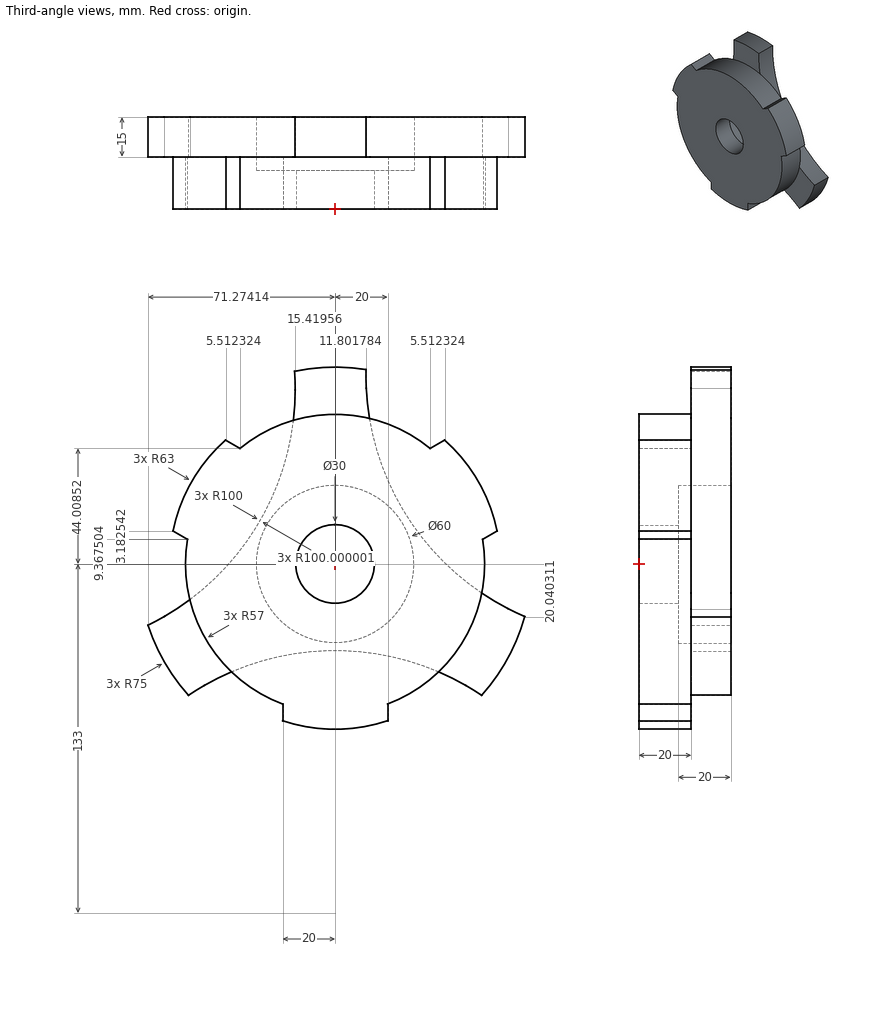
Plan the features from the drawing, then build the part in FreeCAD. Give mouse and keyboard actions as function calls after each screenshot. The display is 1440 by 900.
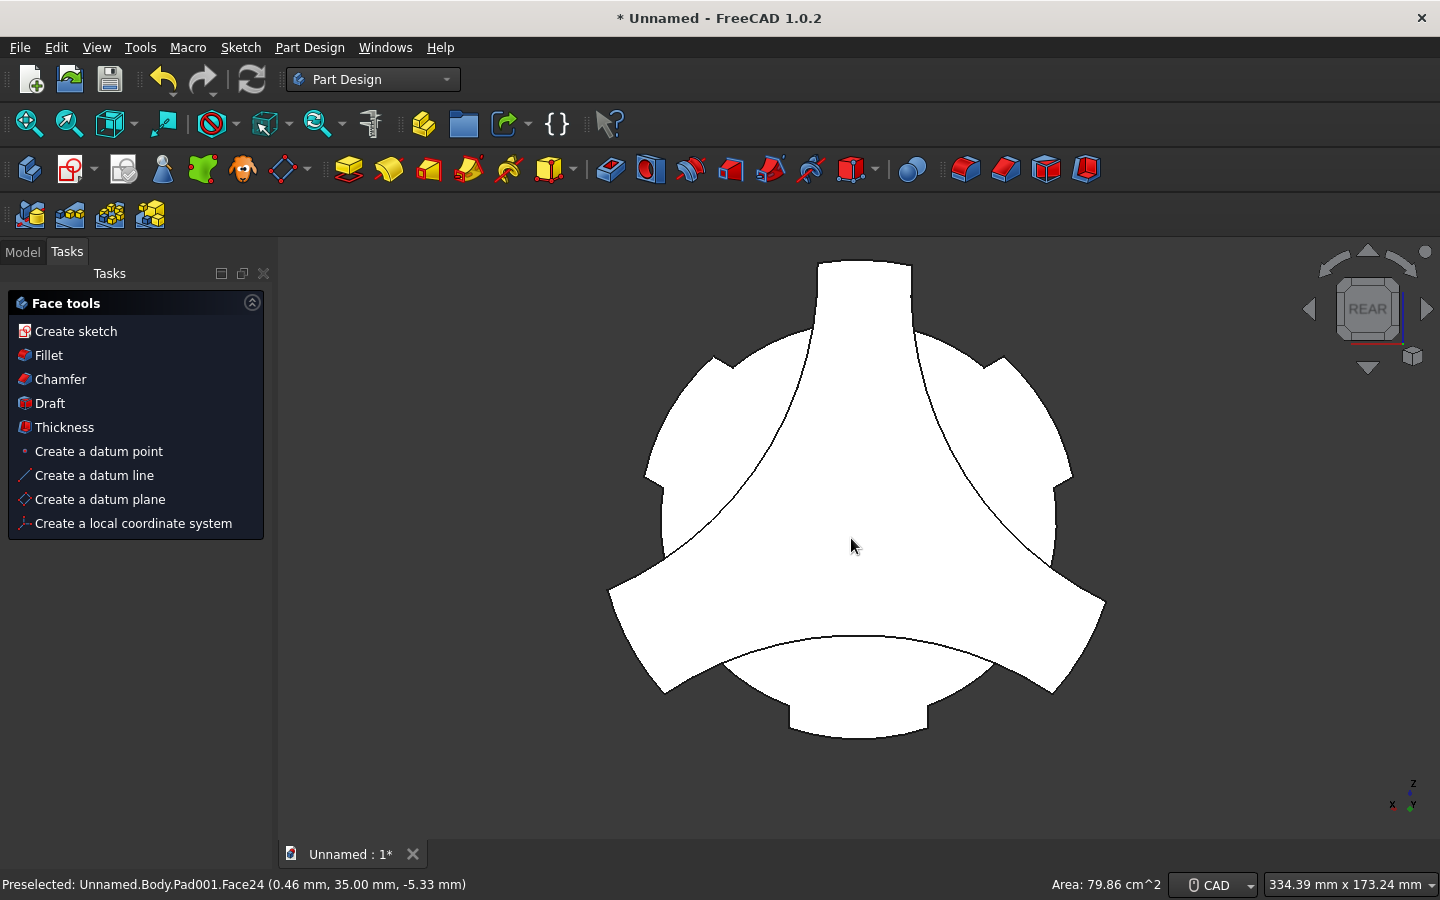
click(70, 170)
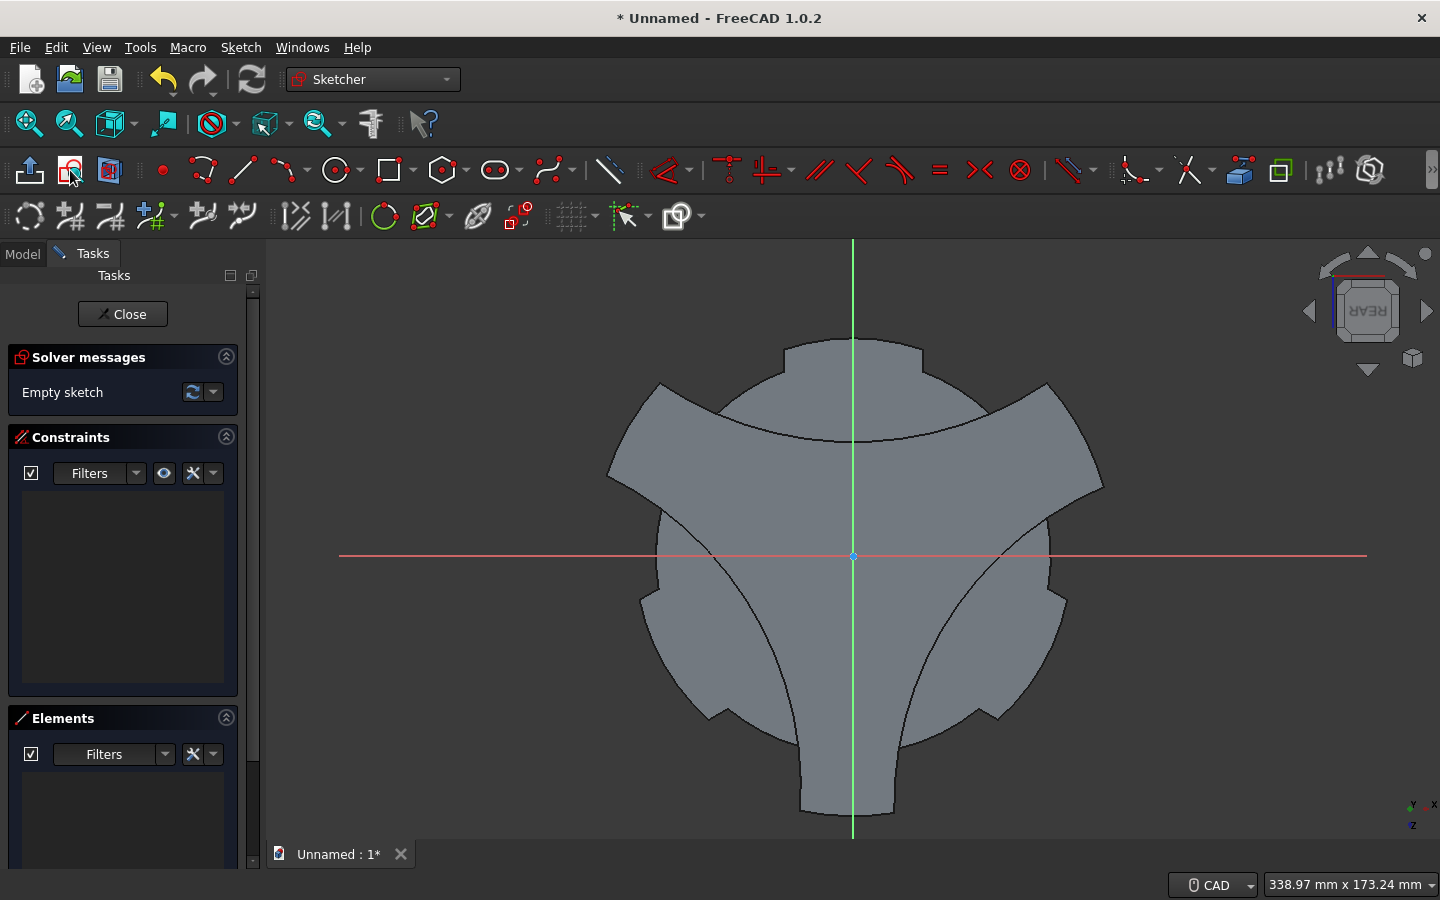
scroll(937, 578, up, 3)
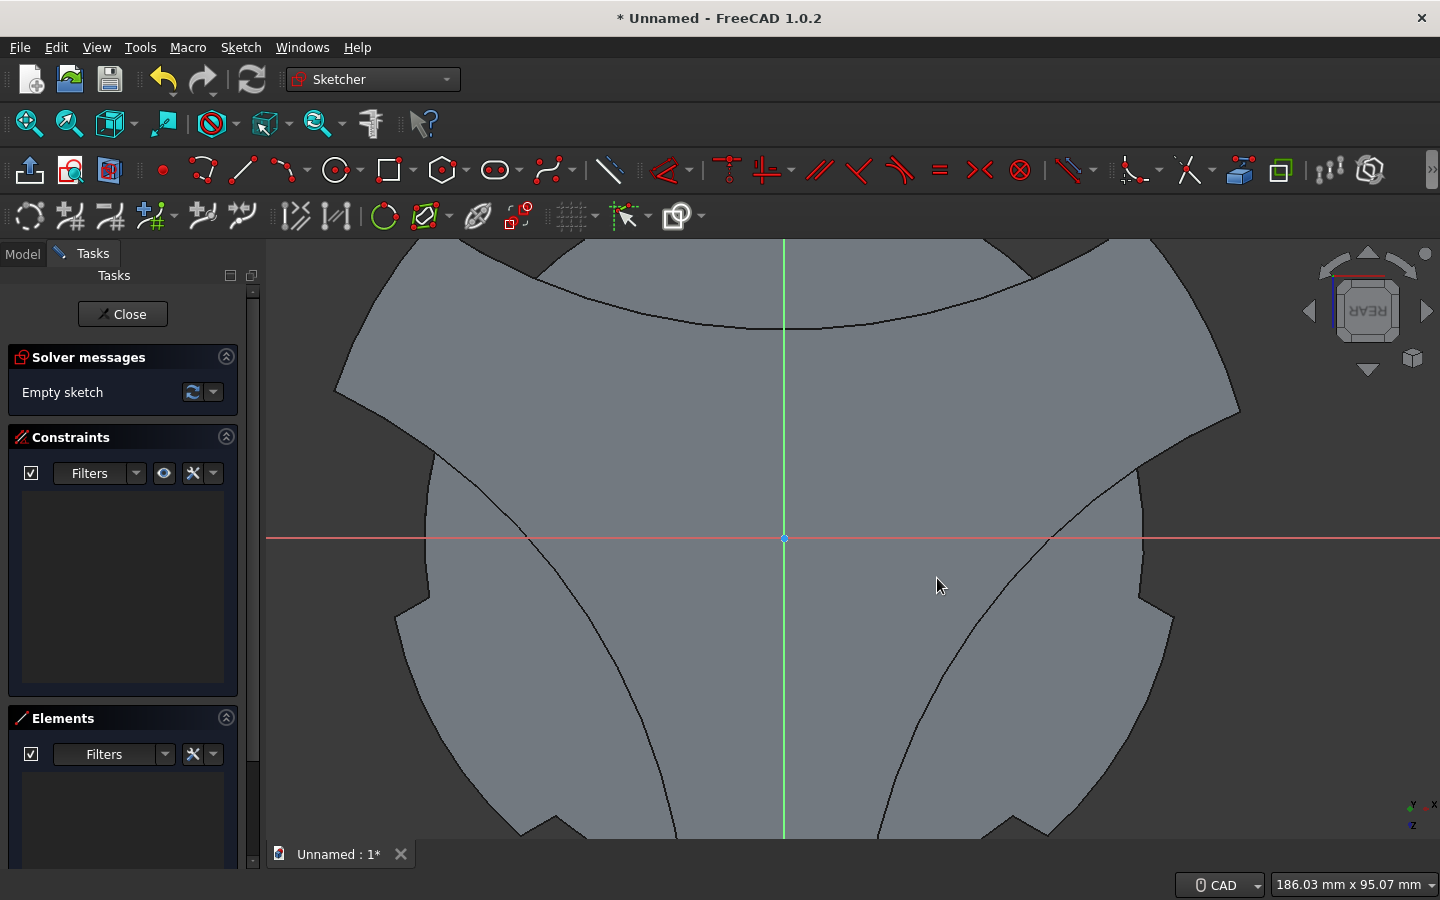
click(336, 170)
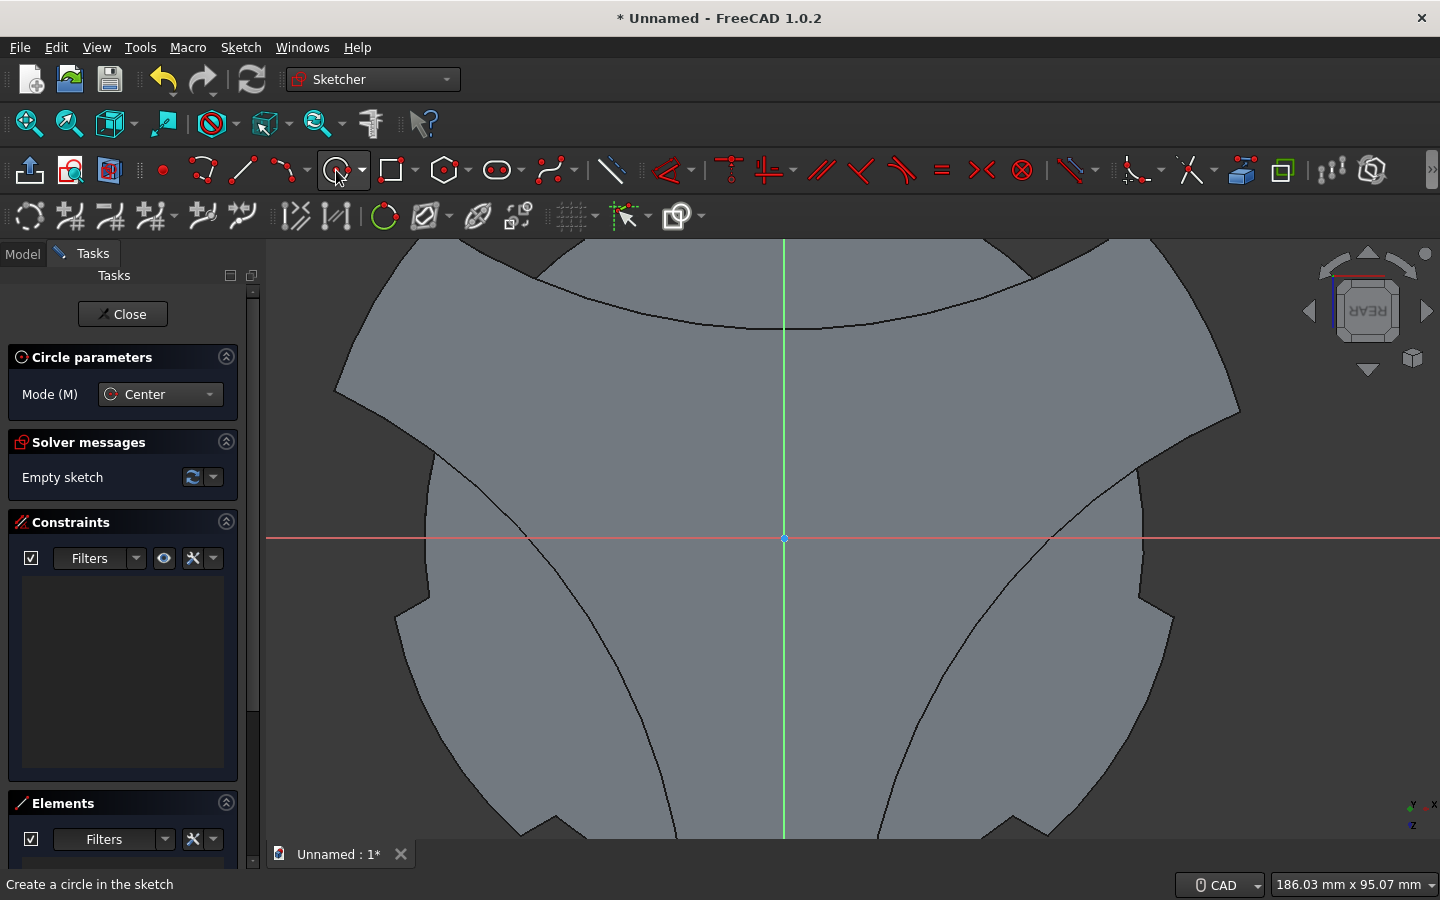
click(784, 538)
move(918, 404)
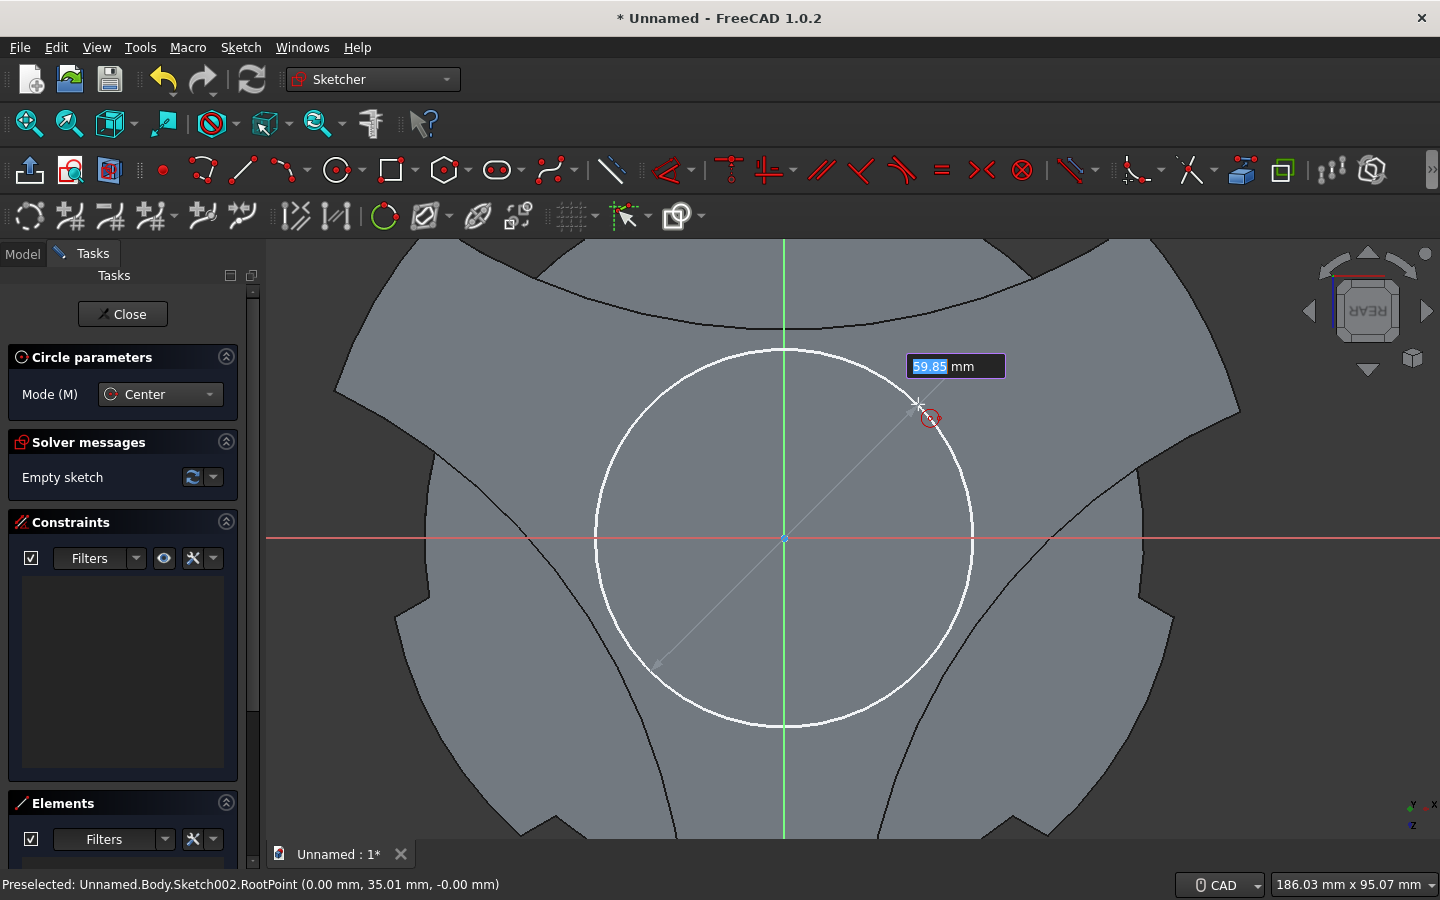
text(60)
key(Return)
key(Escape)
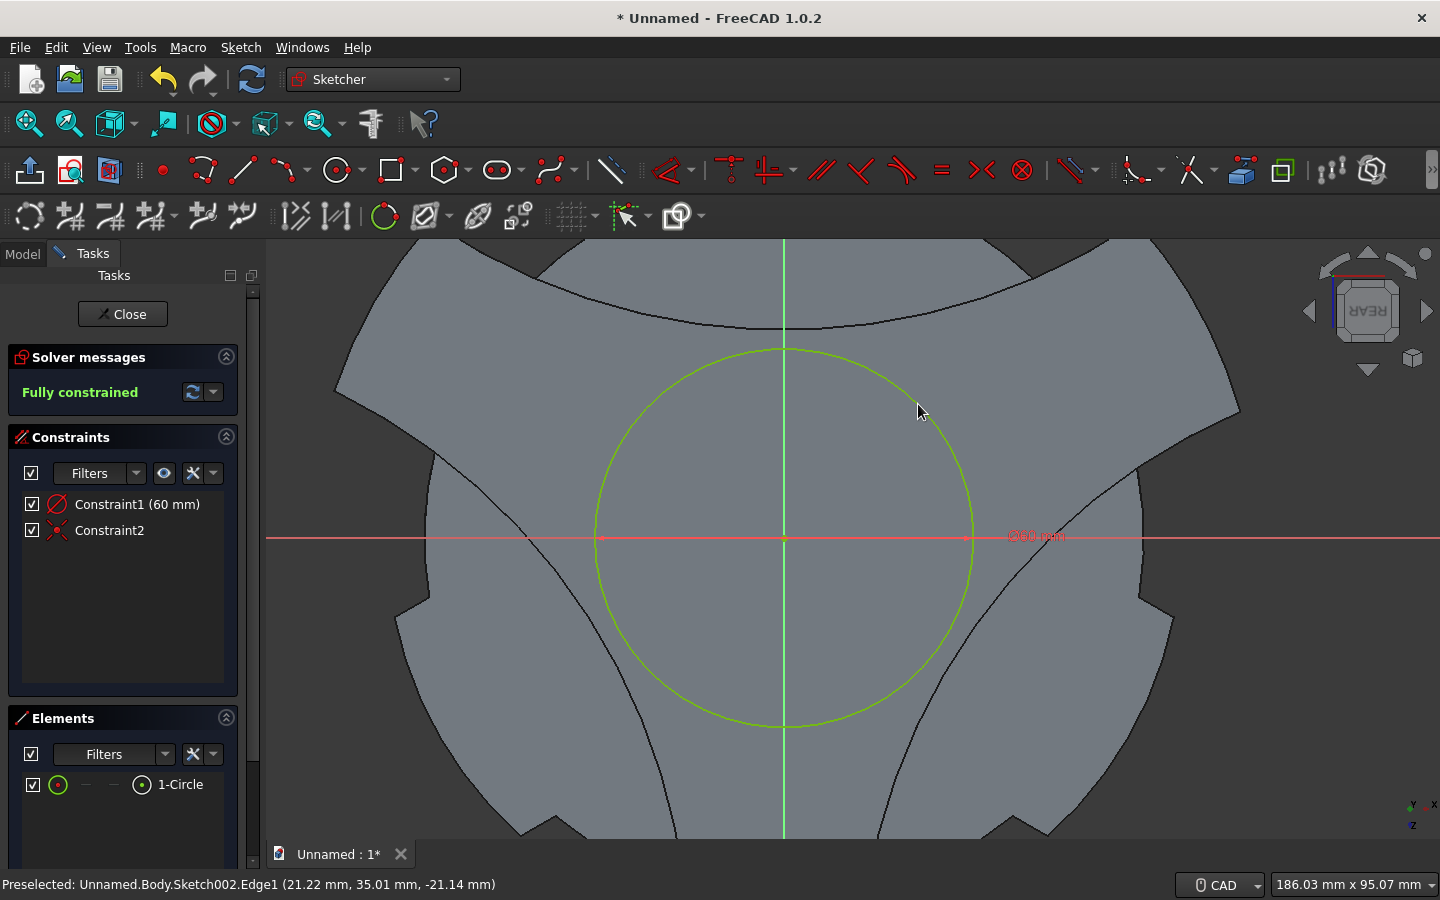
click(123, 314)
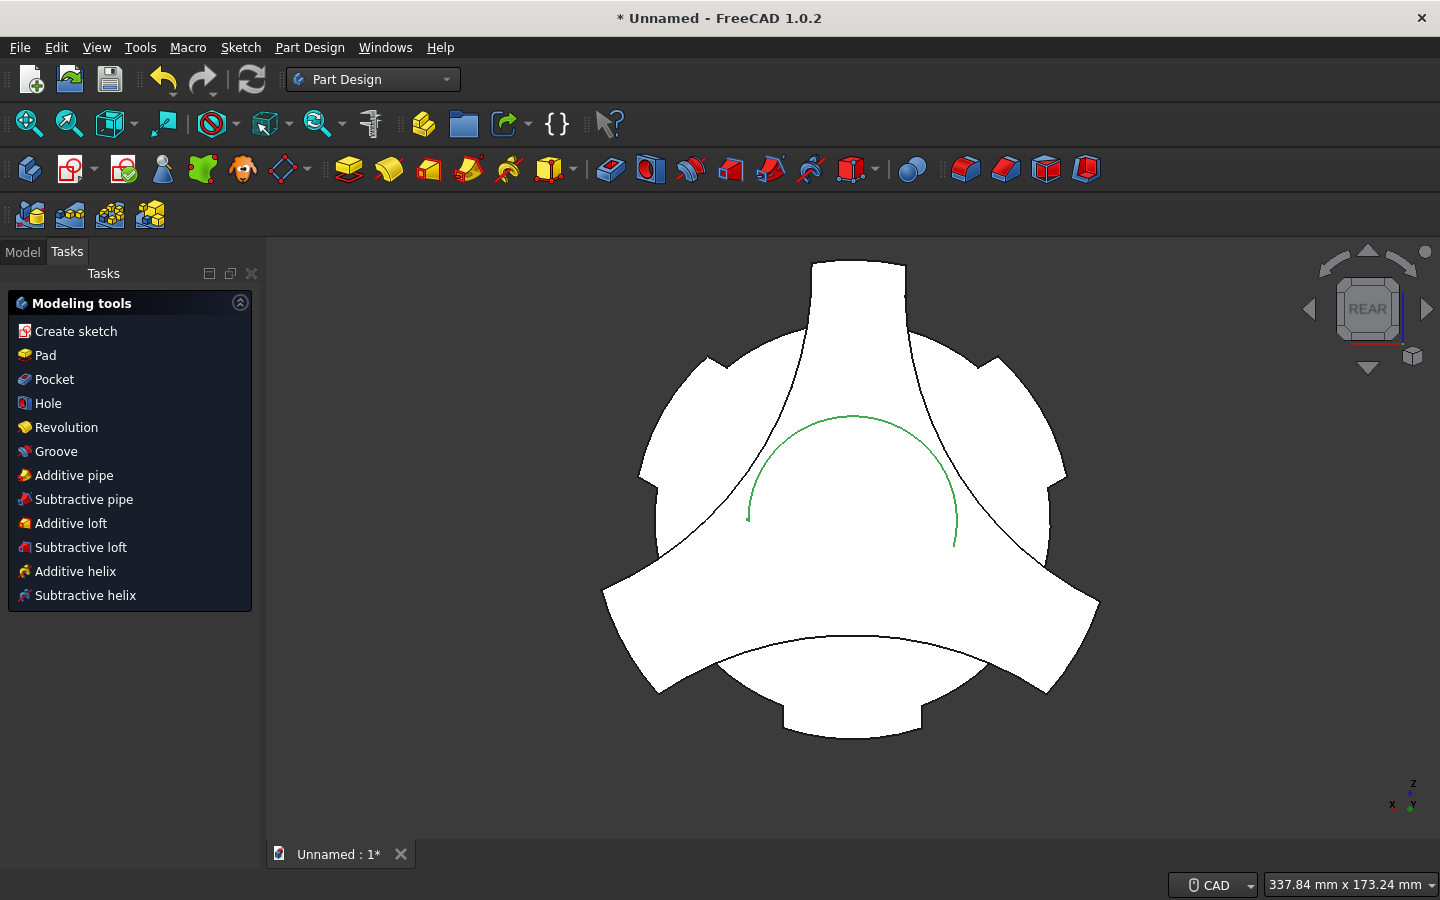
click(612, 170)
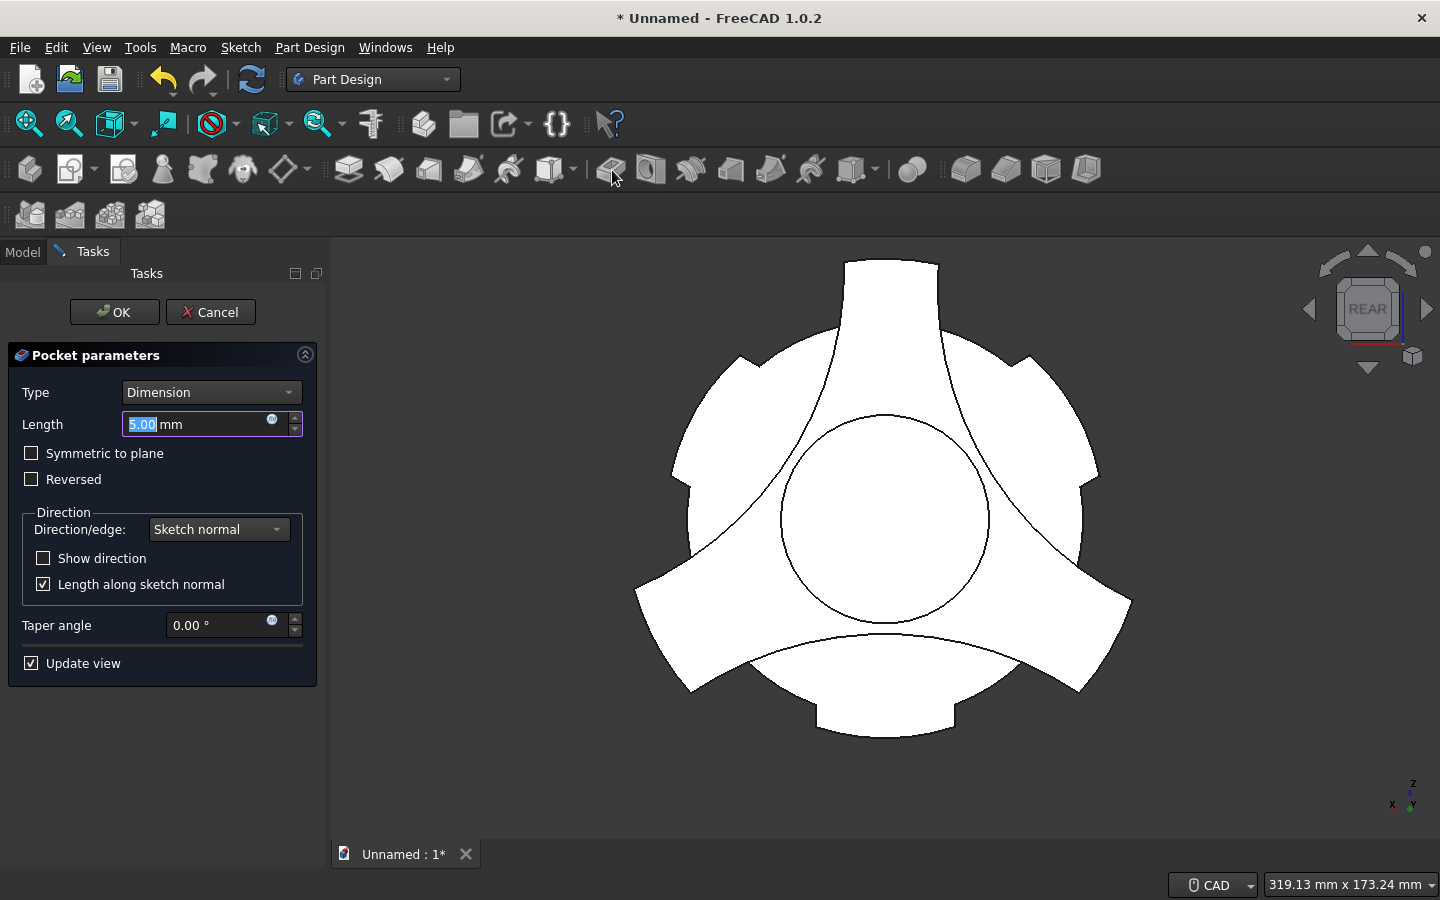
text(20)
key(Tab)